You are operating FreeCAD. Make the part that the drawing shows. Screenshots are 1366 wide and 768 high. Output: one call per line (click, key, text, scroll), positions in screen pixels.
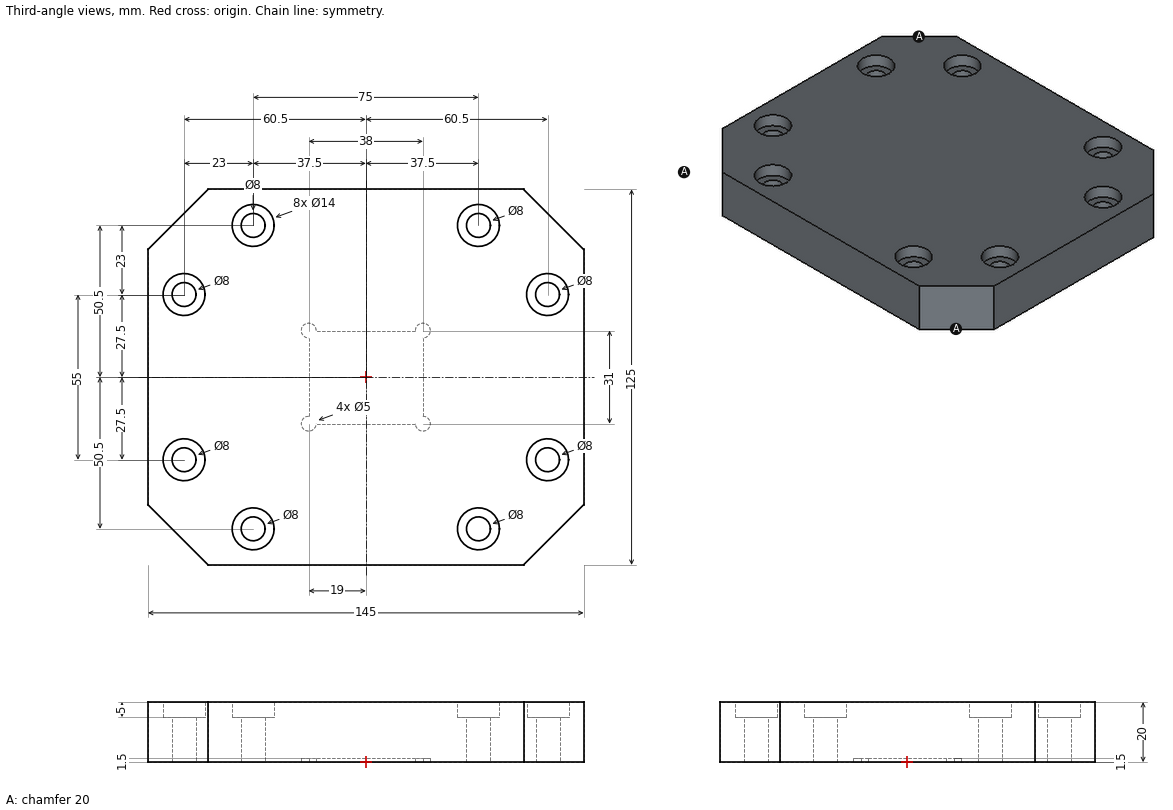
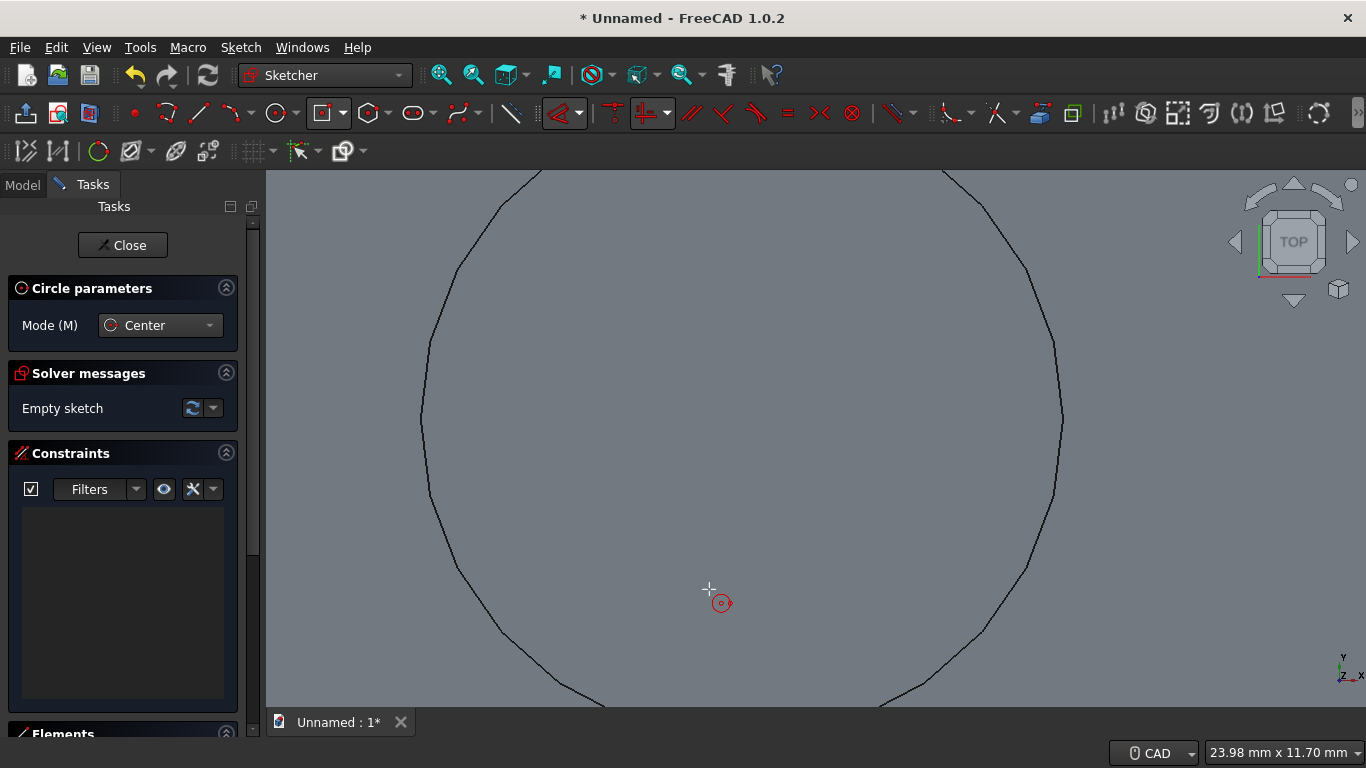
click(742, 419)
click(872, 289)
key(Escape)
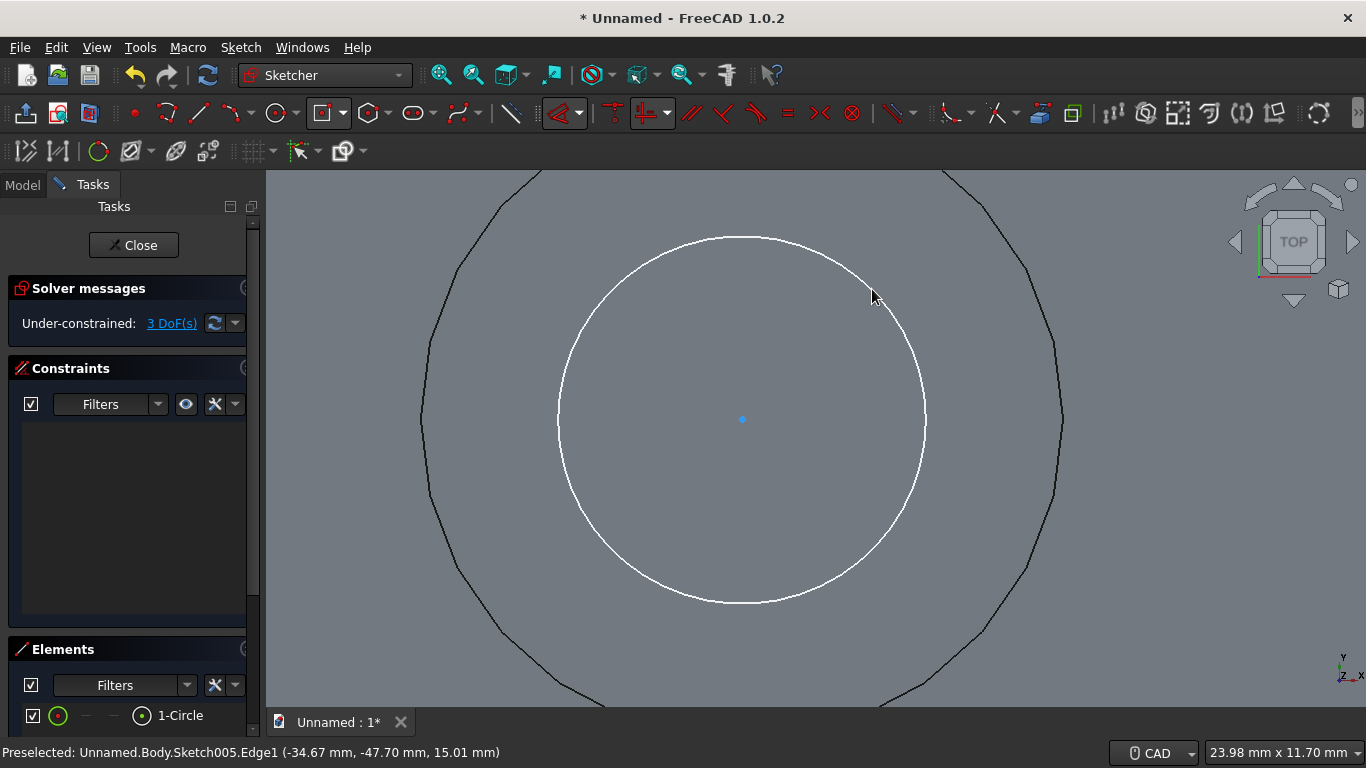
click(872, 290)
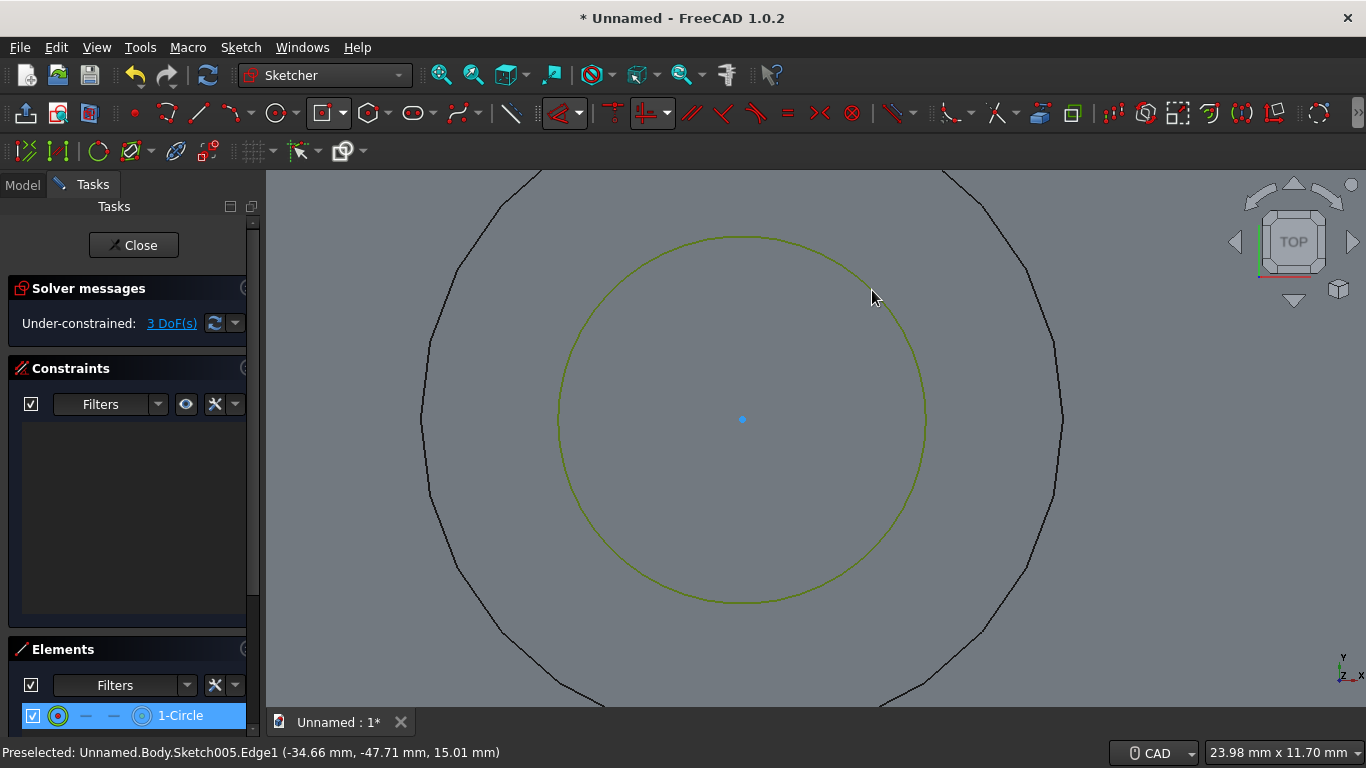
key(k)
key(o)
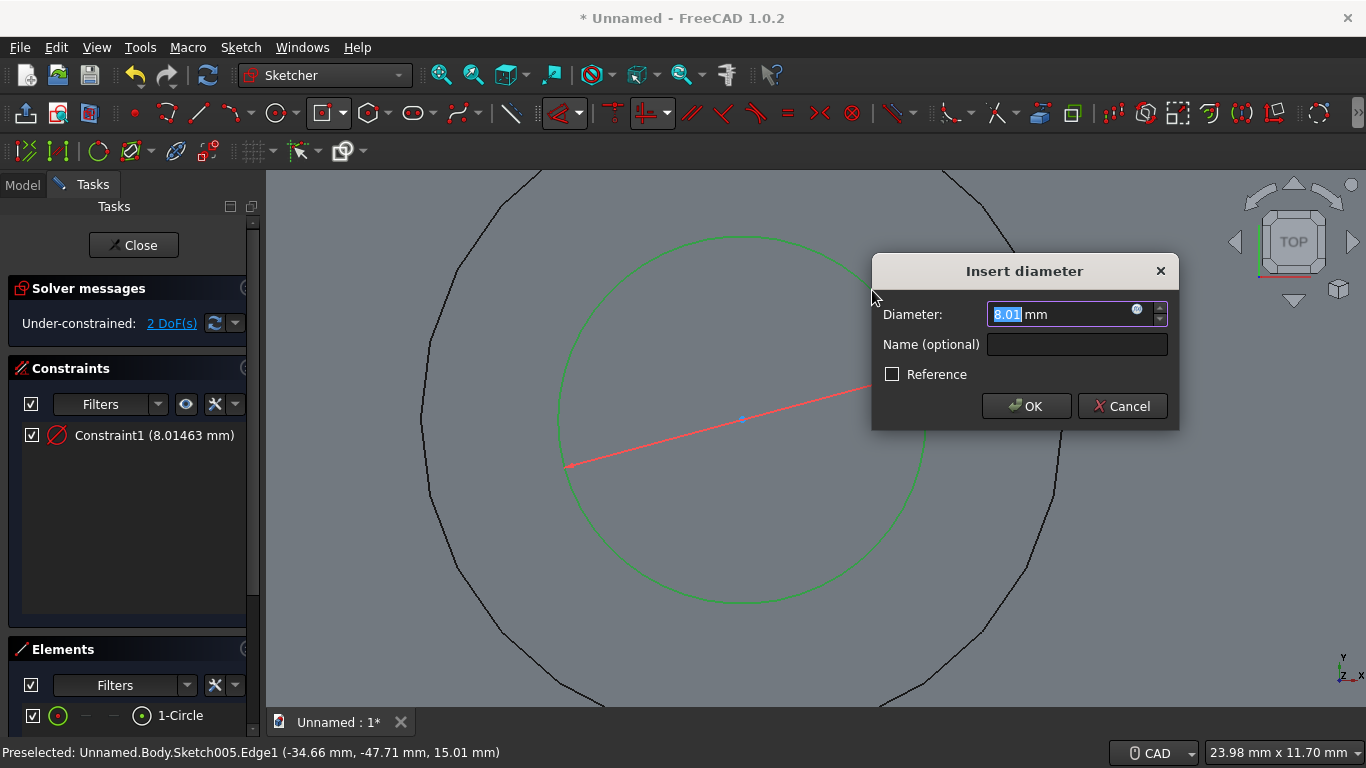
text(8)
key(Return)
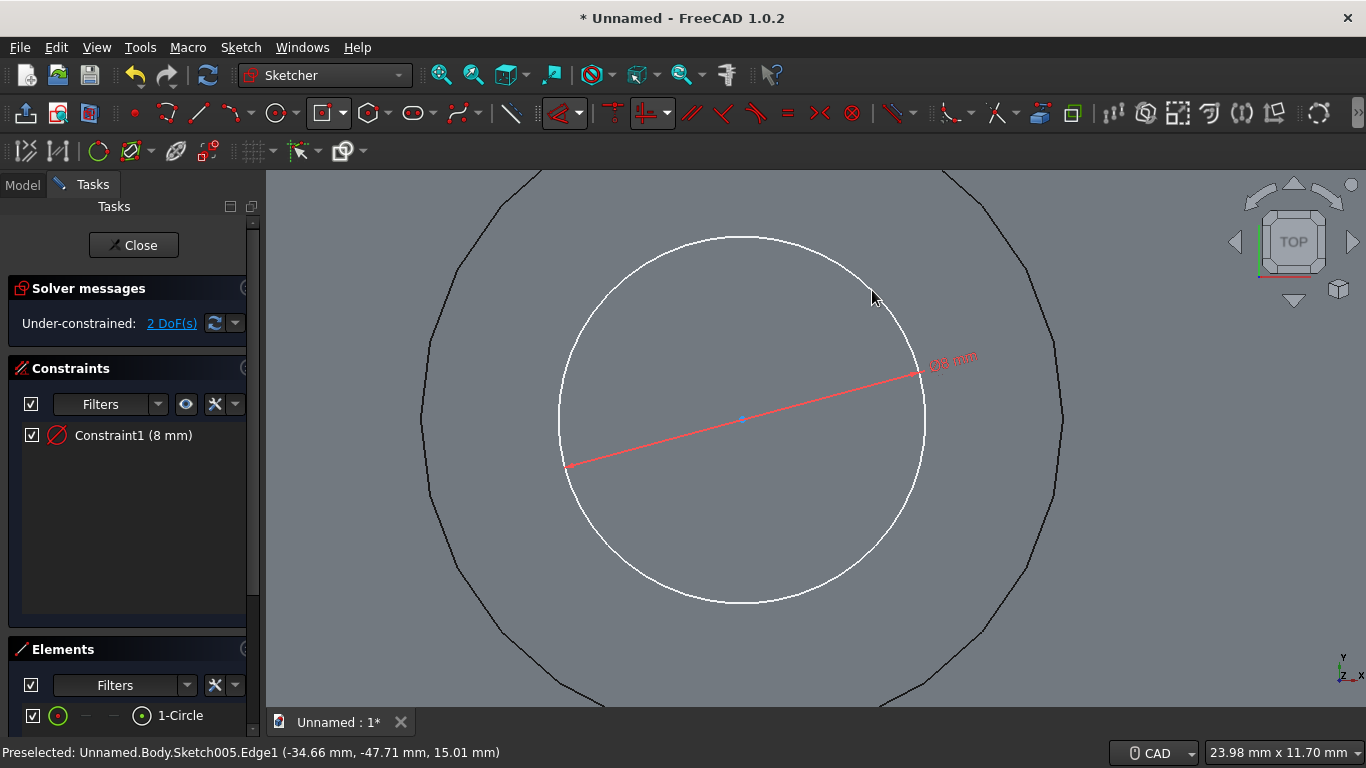
click(742, 420)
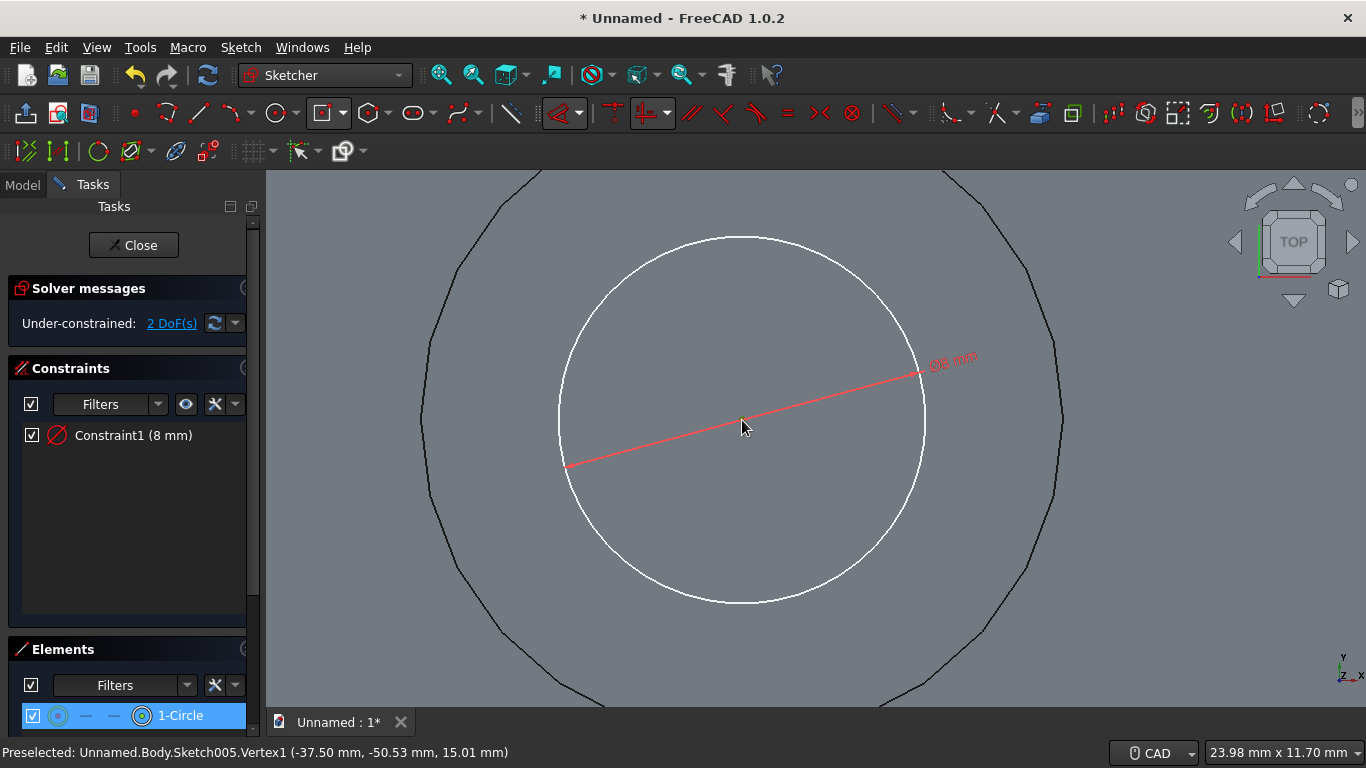
click(582, 114)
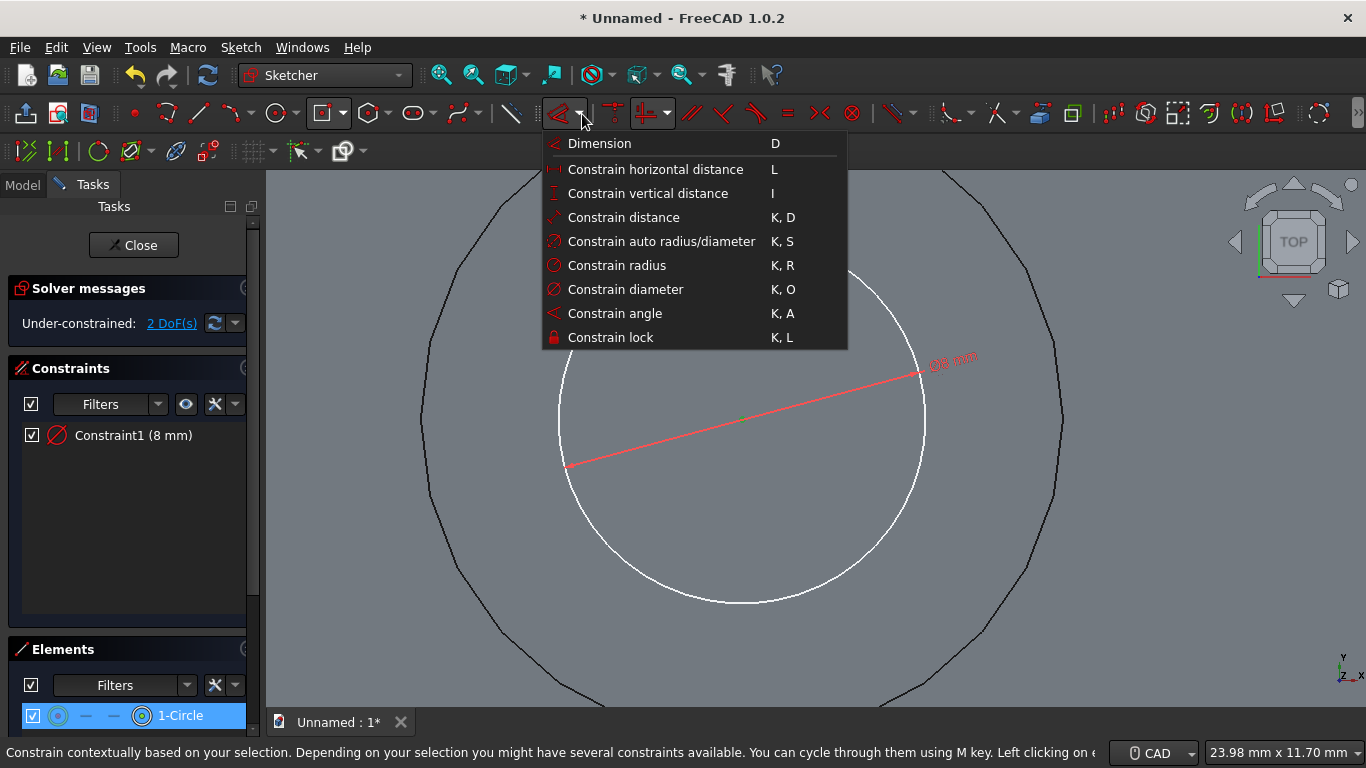
click(695, 169)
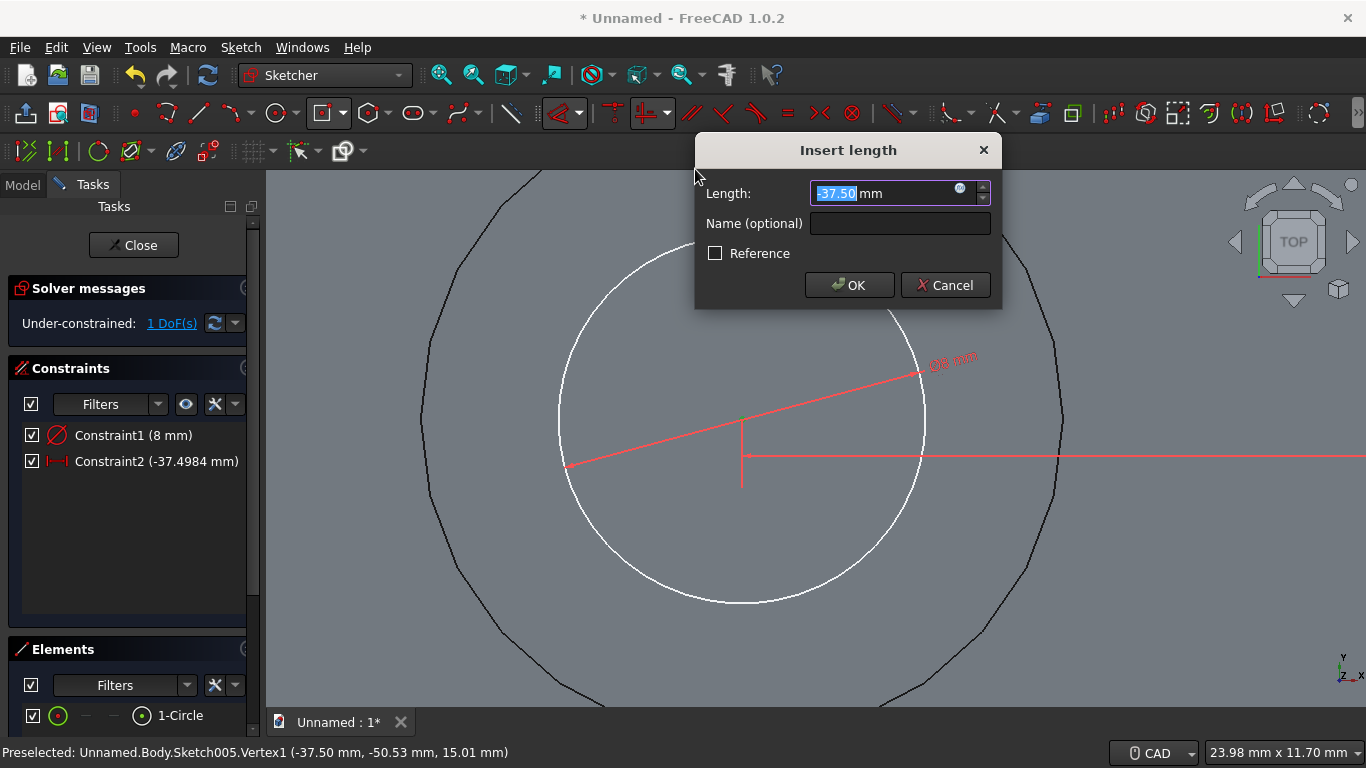
text(-37.5)
key(Return)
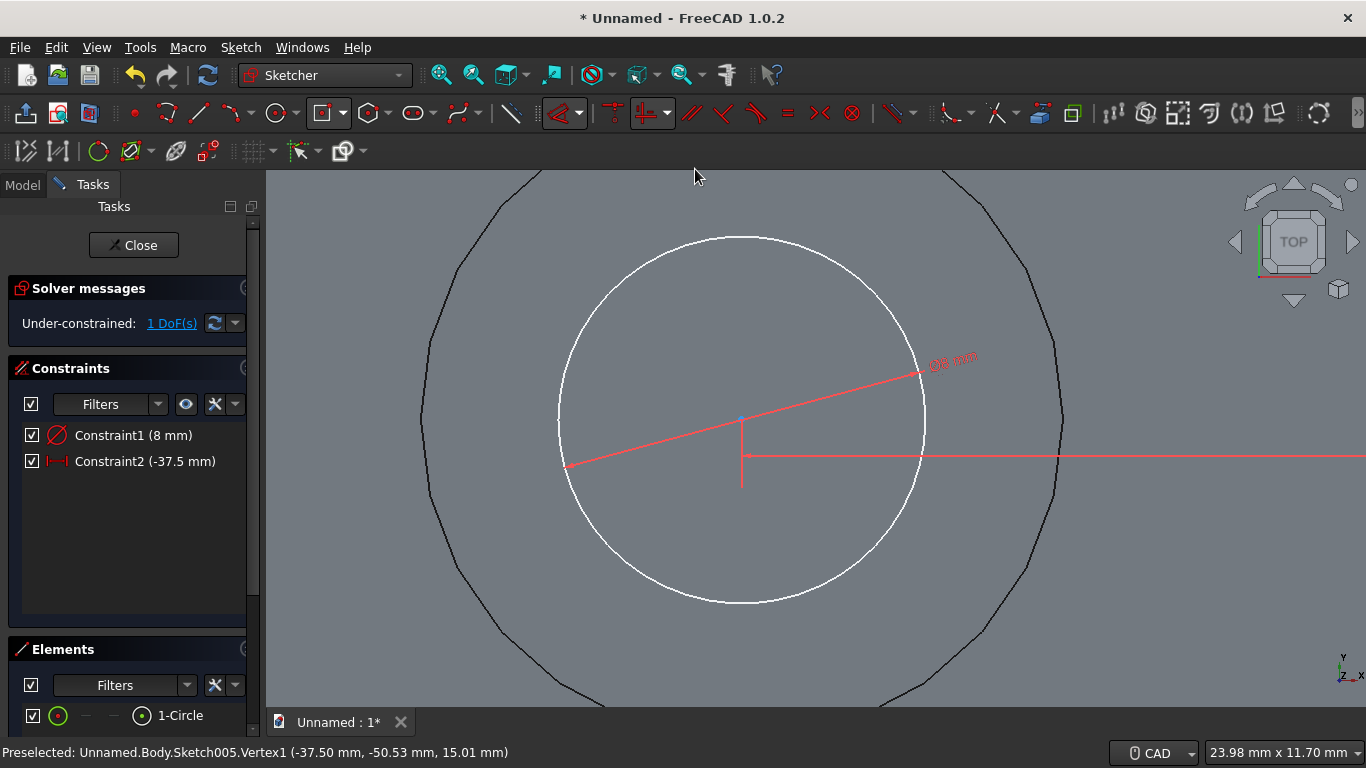
click(742, 420)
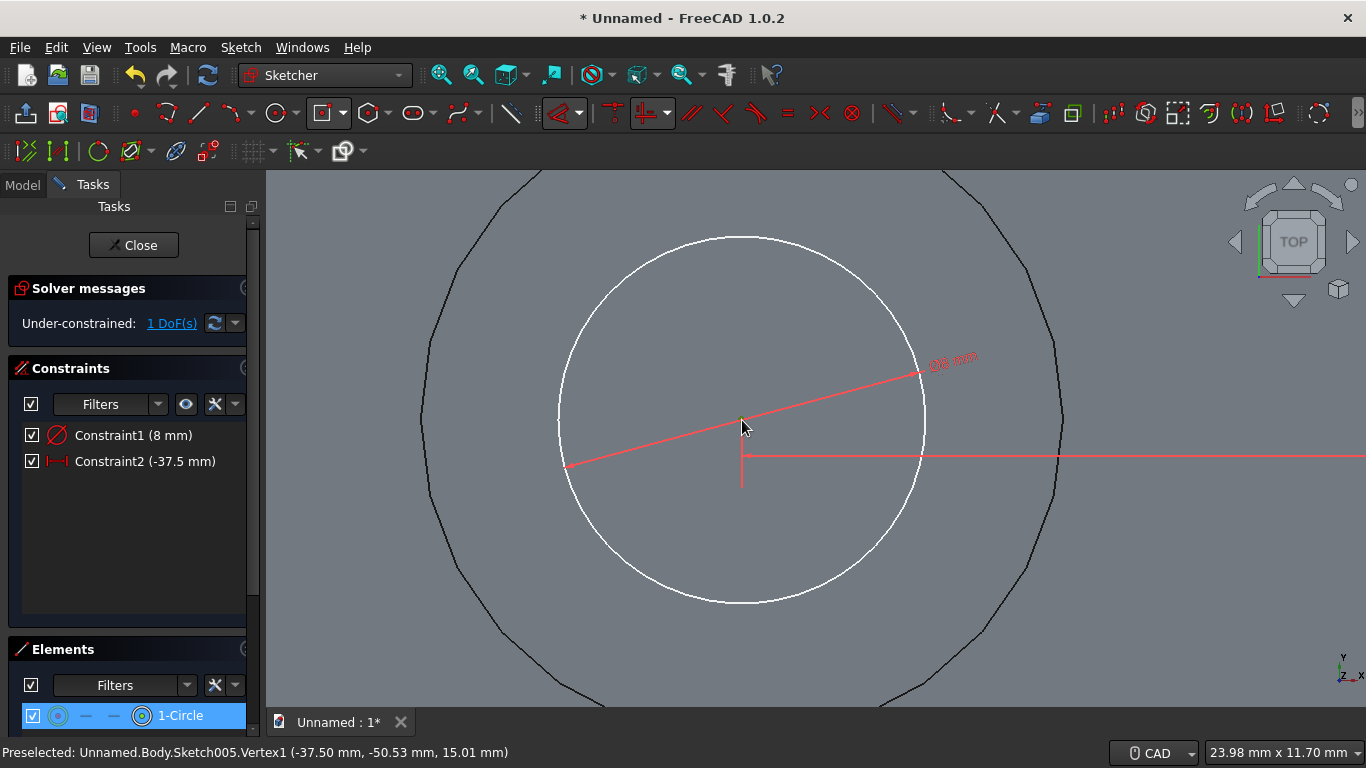
key(i)